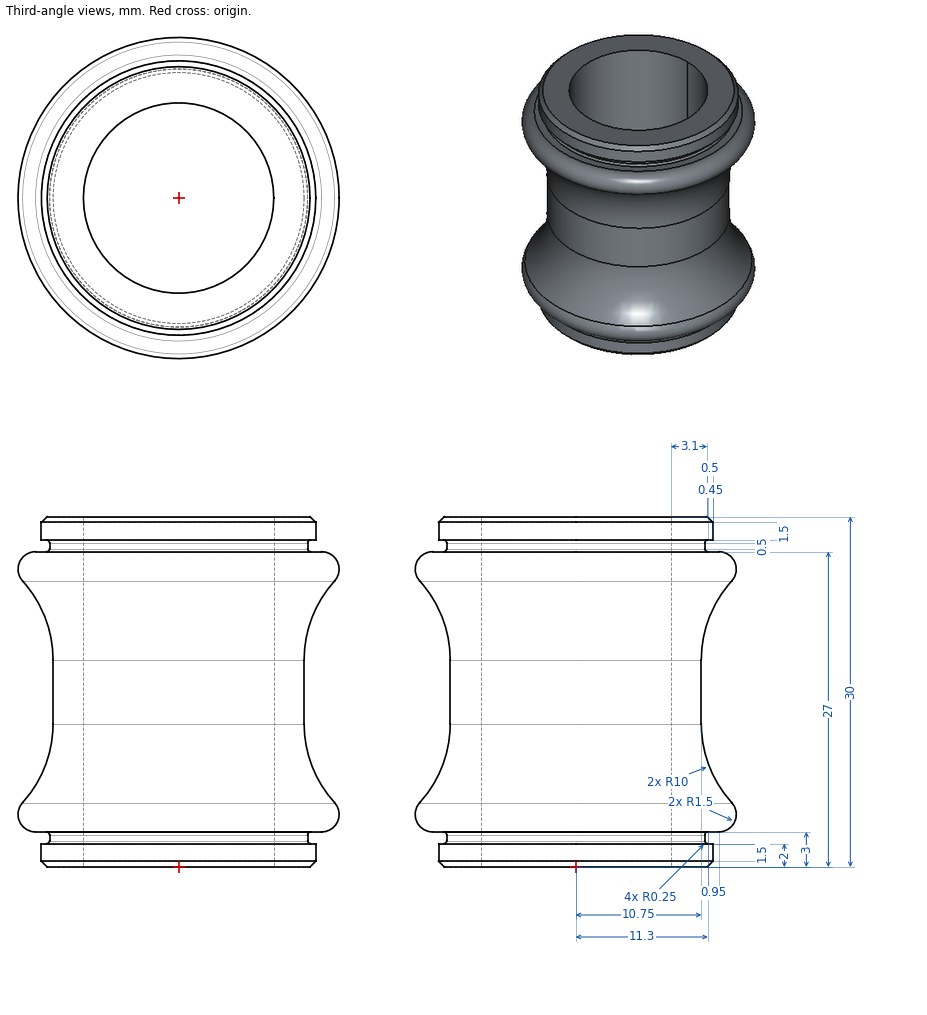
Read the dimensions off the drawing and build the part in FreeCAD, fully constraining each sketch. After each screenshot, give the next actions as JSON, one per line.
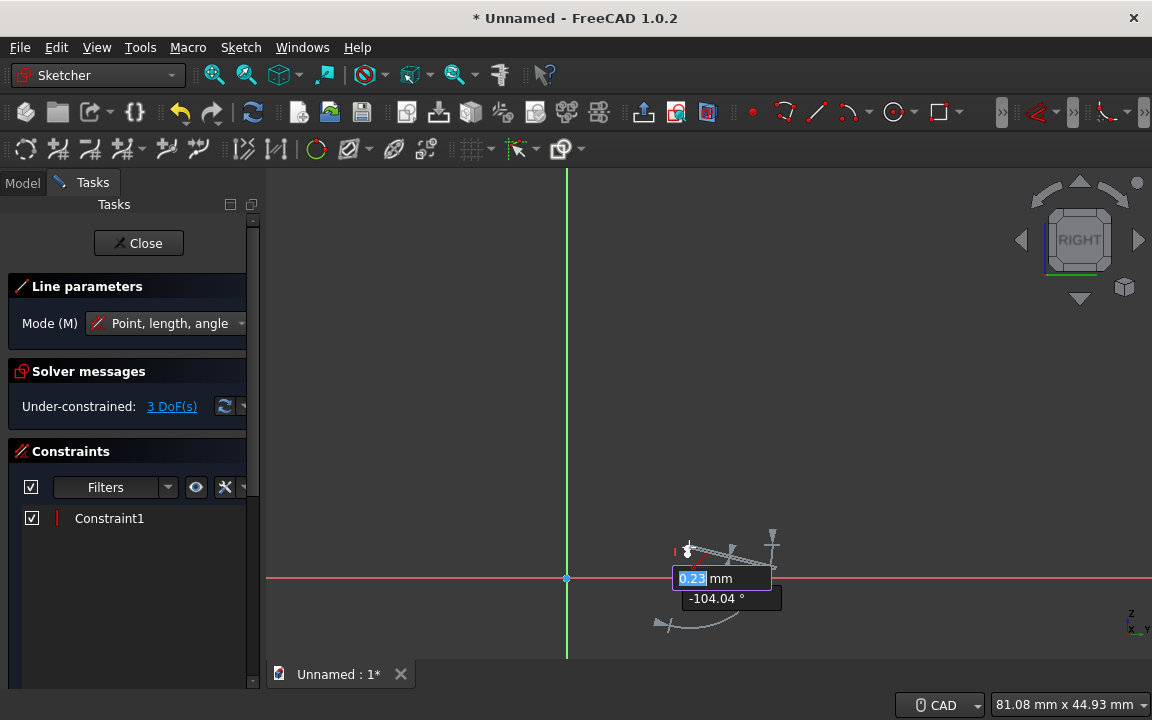
{"action": "scroll", "coordinate": [700, 545], "scroll_direction": "up", "scroll_amount": 3}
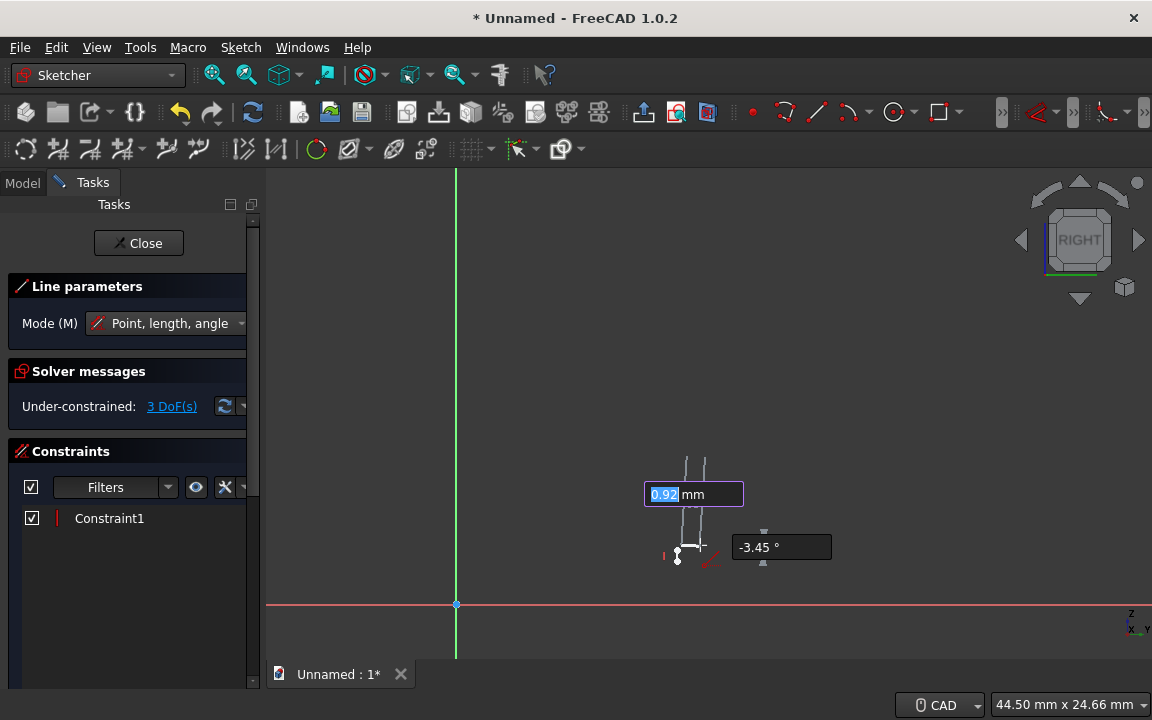
{"action": "left_click", "coordinate": [700, 545]}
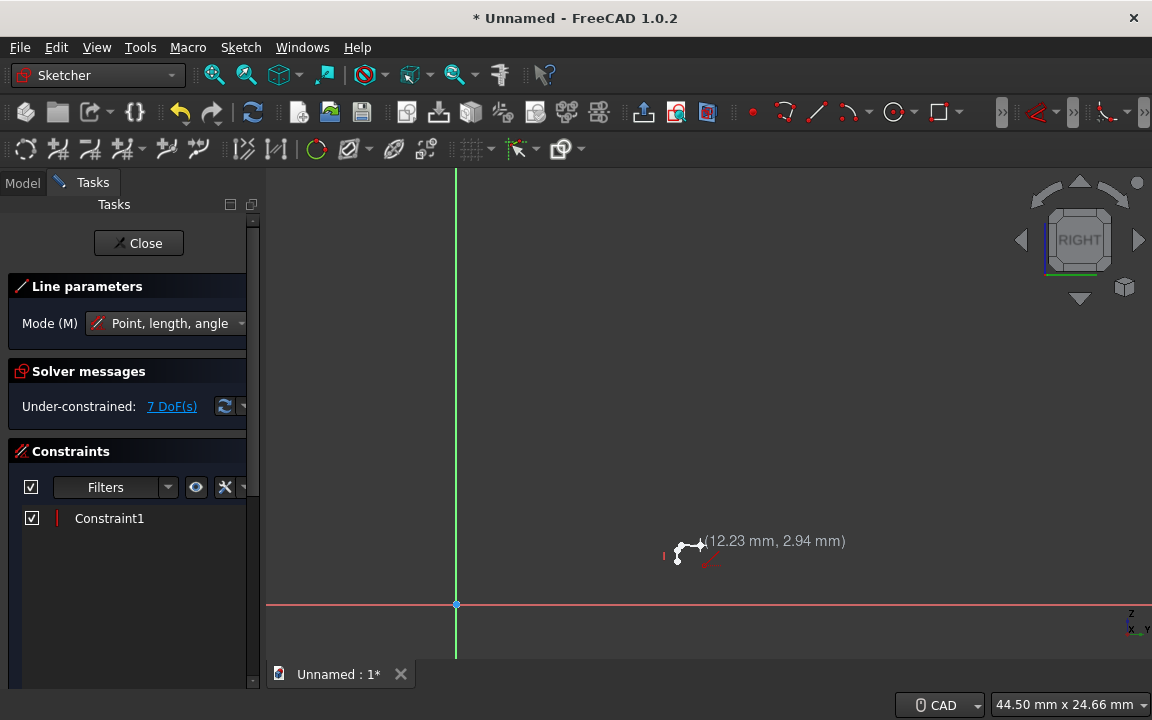
{"action": "left_click", "coordinate": [670, 361]}
{"action": "left_click", "coordinate": [670, 251]}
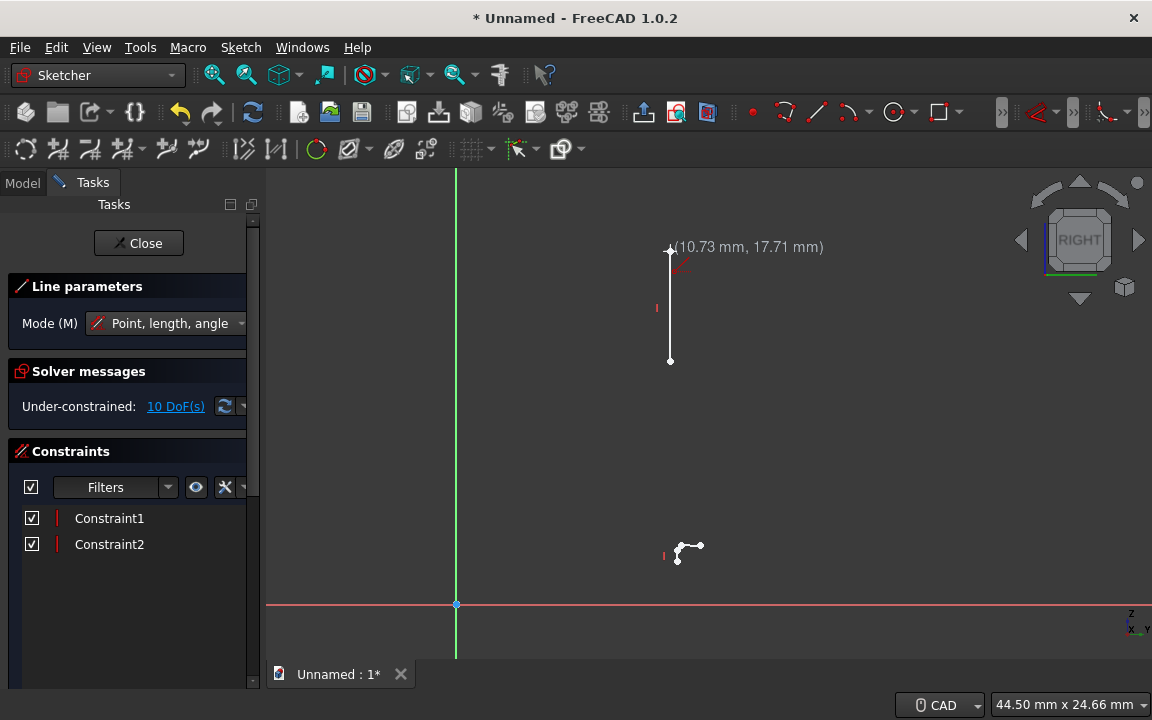
{"action": "scroll", "coordinate": [699, 544], "scroll_direction": "down", "scroll_amount": 3}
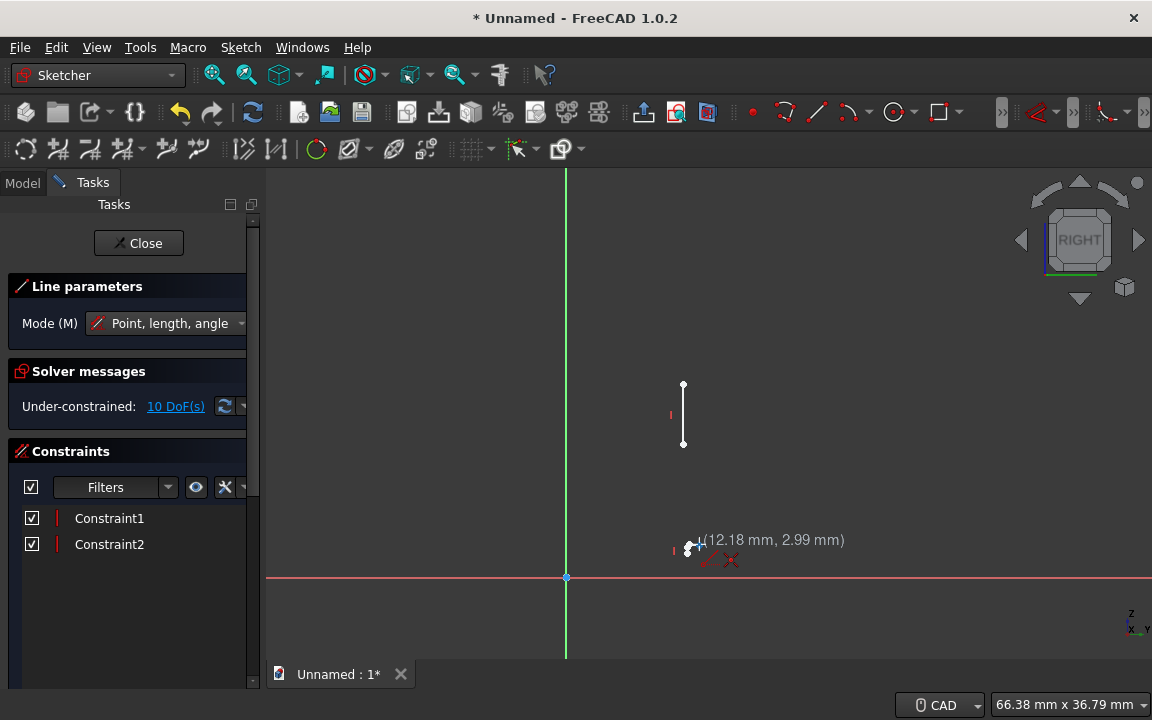
{"action": "left_click", "coordinate": [700, 283]}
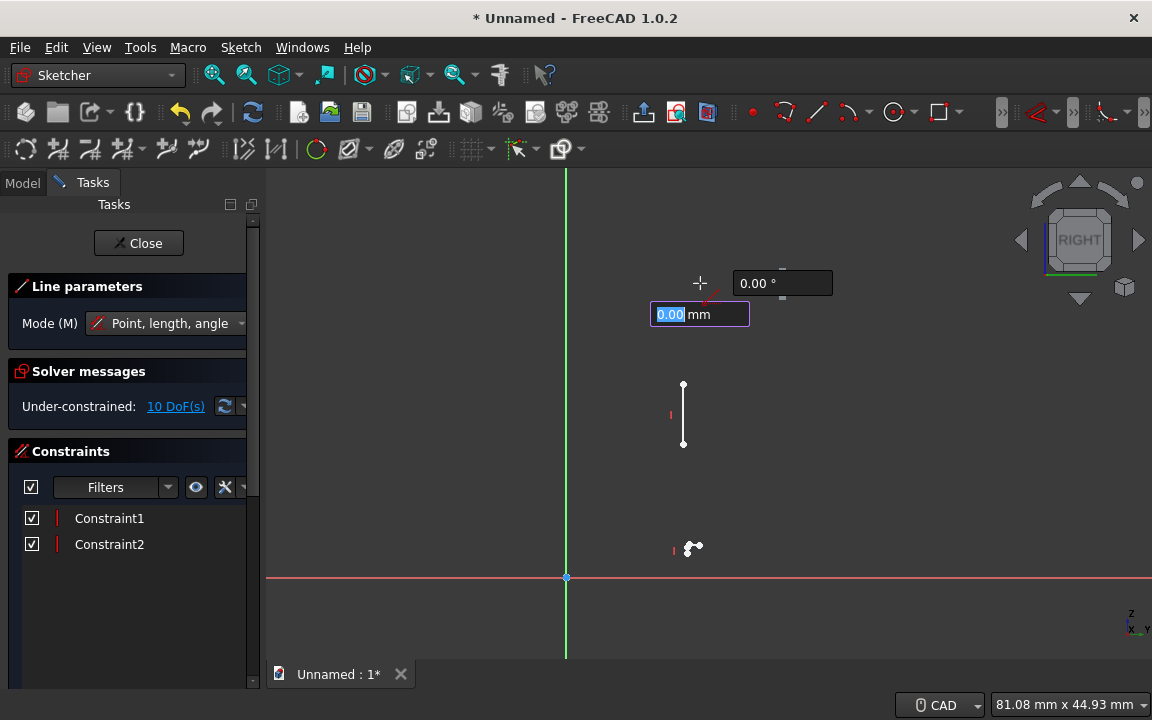
{"action": "scroll", "coordinate": [690, 283], "scroll_direction": "up", "scroll_amount": 3}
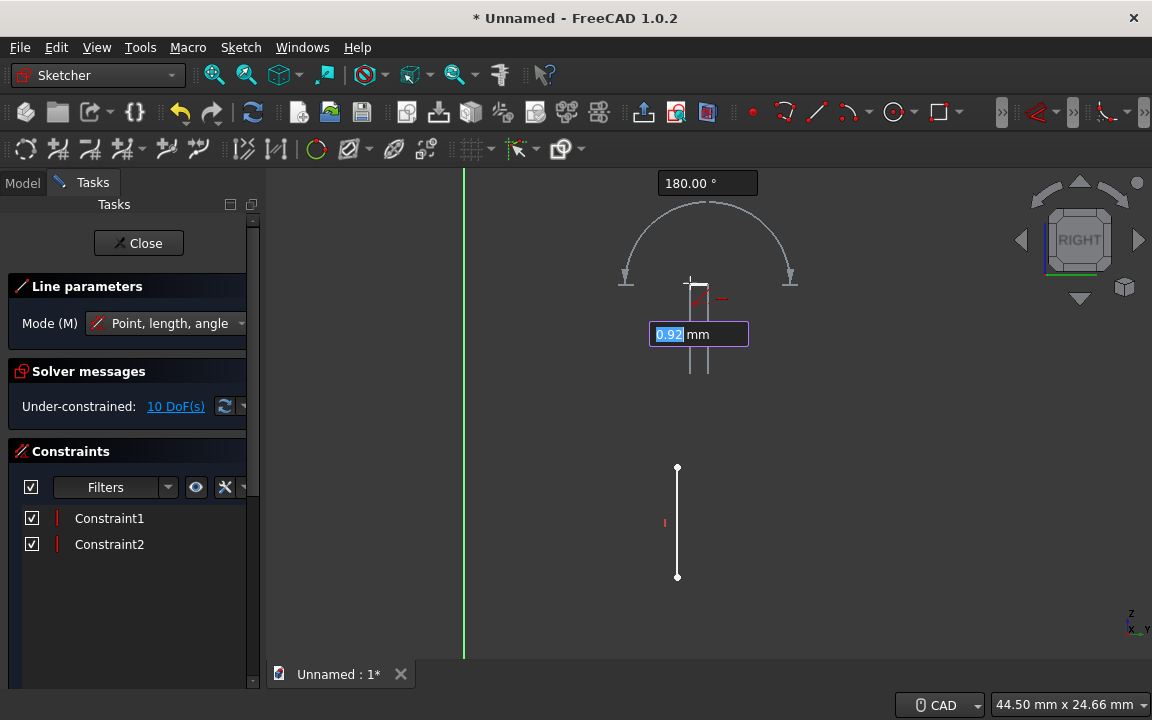
{"action": "left_click", "coordinate": [689, 283]}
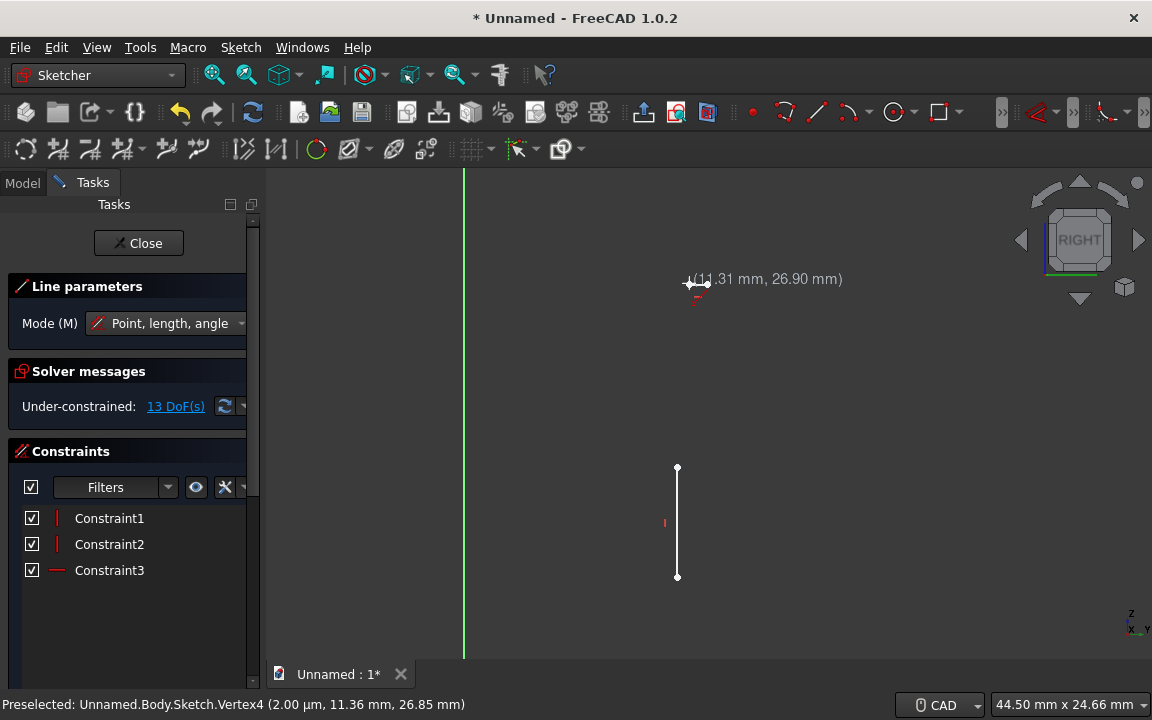
{"action": "scroll", "coordinate": [684, 277], "scroll_direction": "up", "scroll_amount": 5}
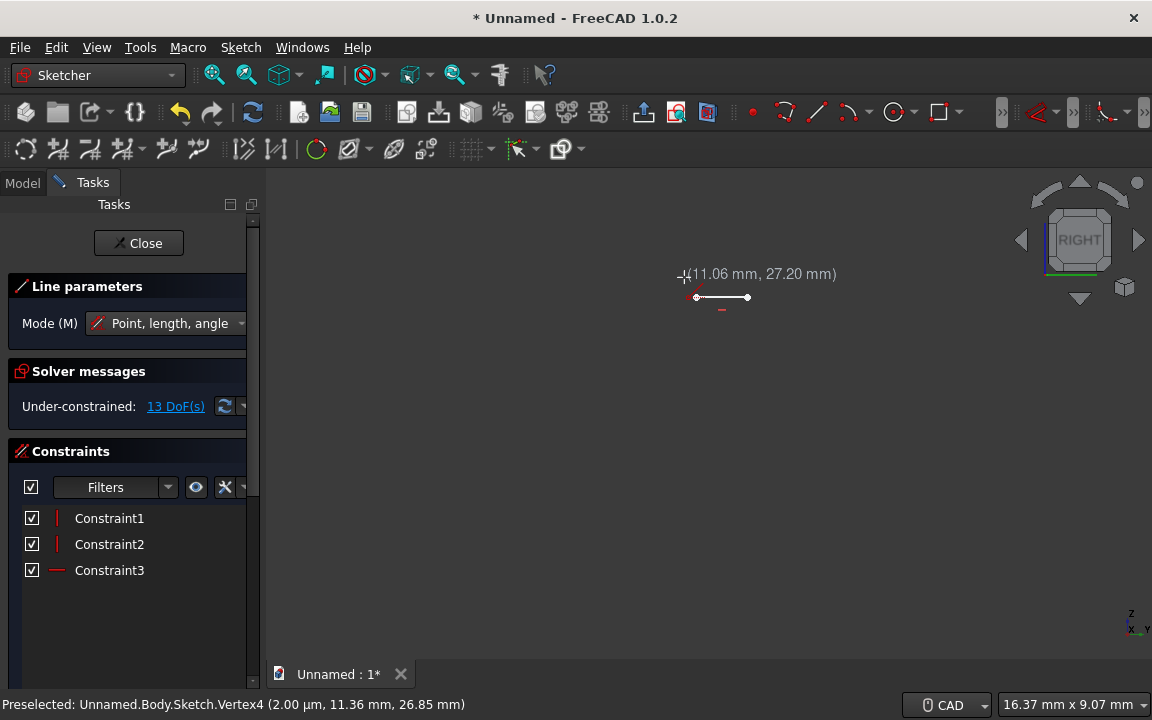
{"action": "left_click", "coordinate": [683, 277]}
{"action": "left_click", "coordinate": [683, 249]}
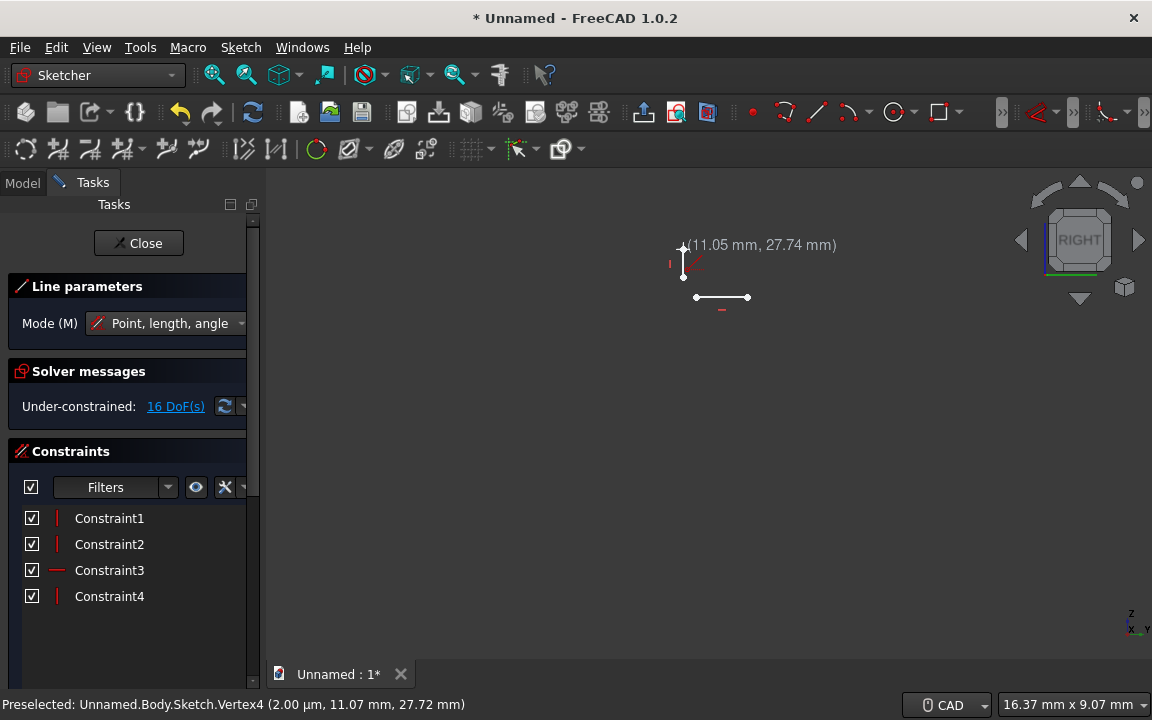
{"action": "key", "text": "g m"}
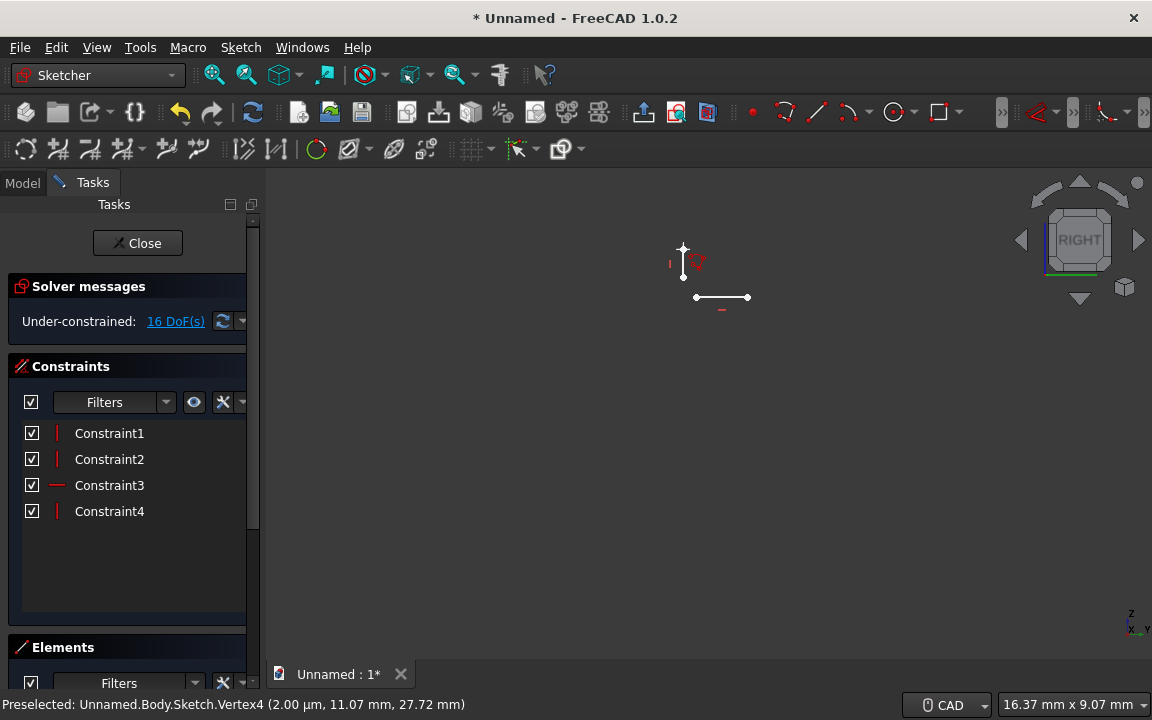
{"action": "left_click", "coordinate": [696, 236]}
{"action": "left_click", "coordinate": [721, 236]}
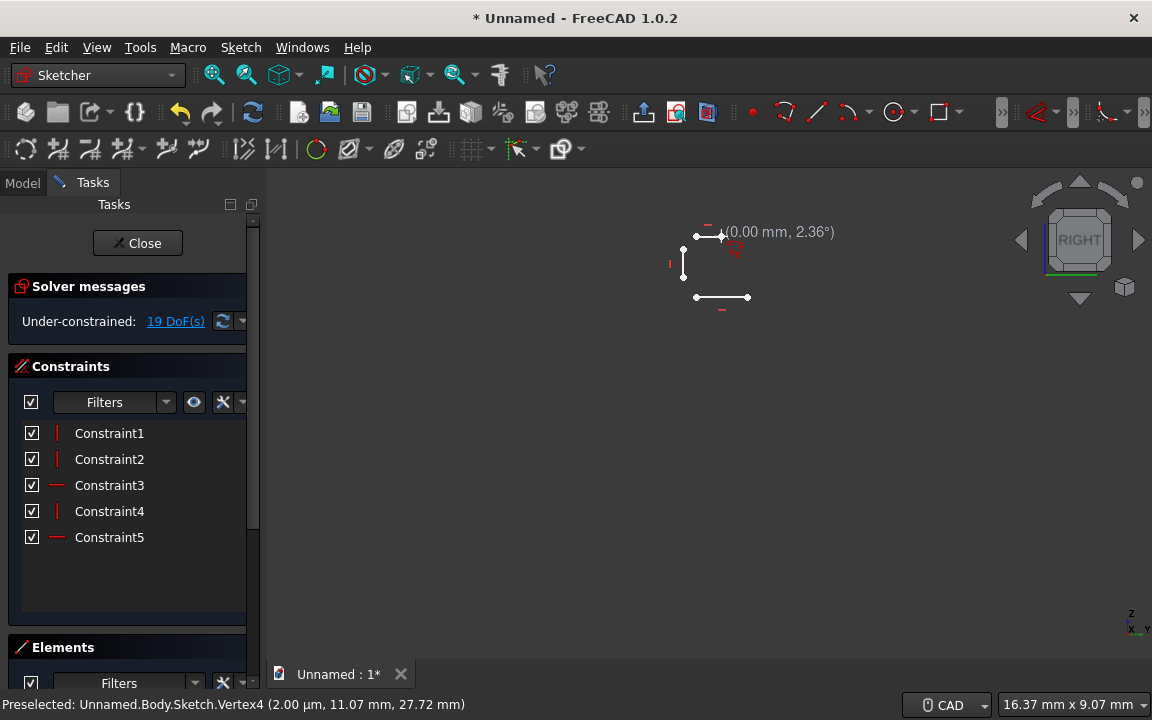
{"action": "scroll", "coordinate": [688, 280], "scroll_direction": "down", "scroll_amount": 8}